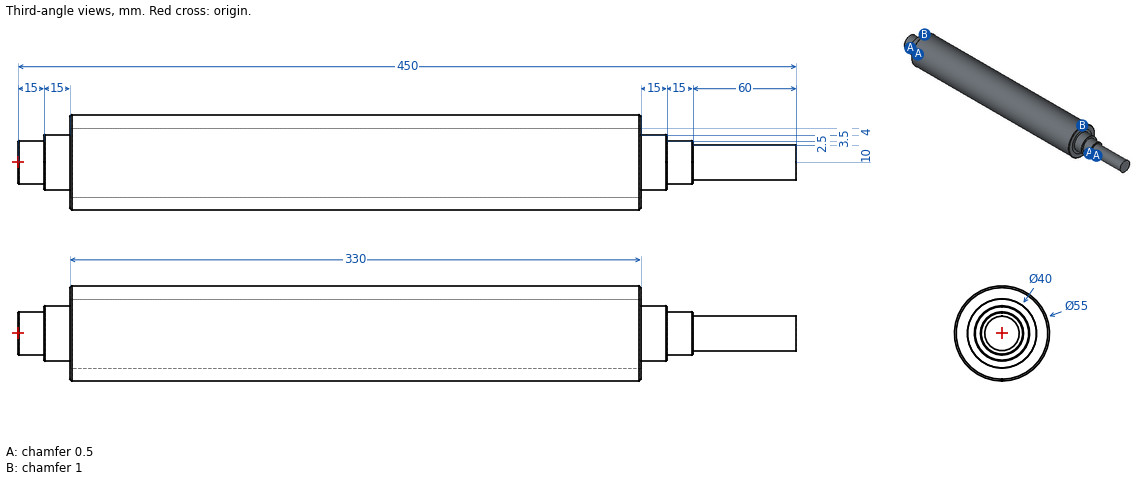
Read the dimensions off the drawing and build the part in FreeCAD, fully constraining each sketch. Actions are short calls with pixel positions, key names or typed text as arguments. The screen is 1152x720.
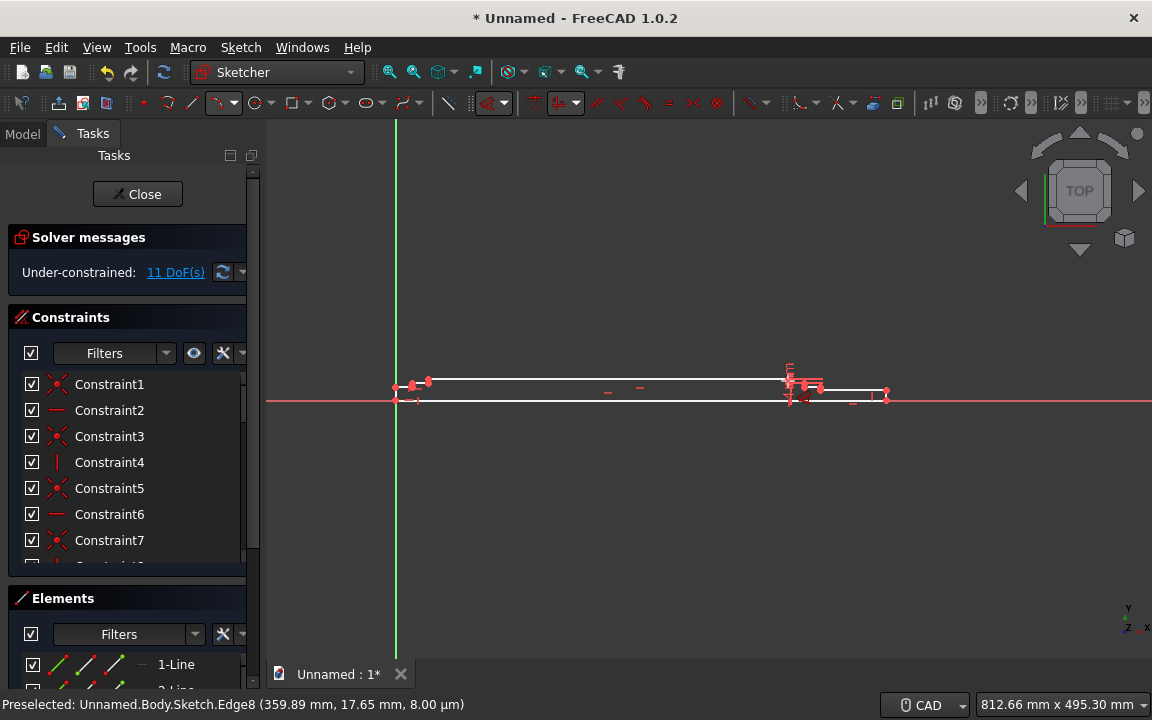
scroll(428, 380, up, 12)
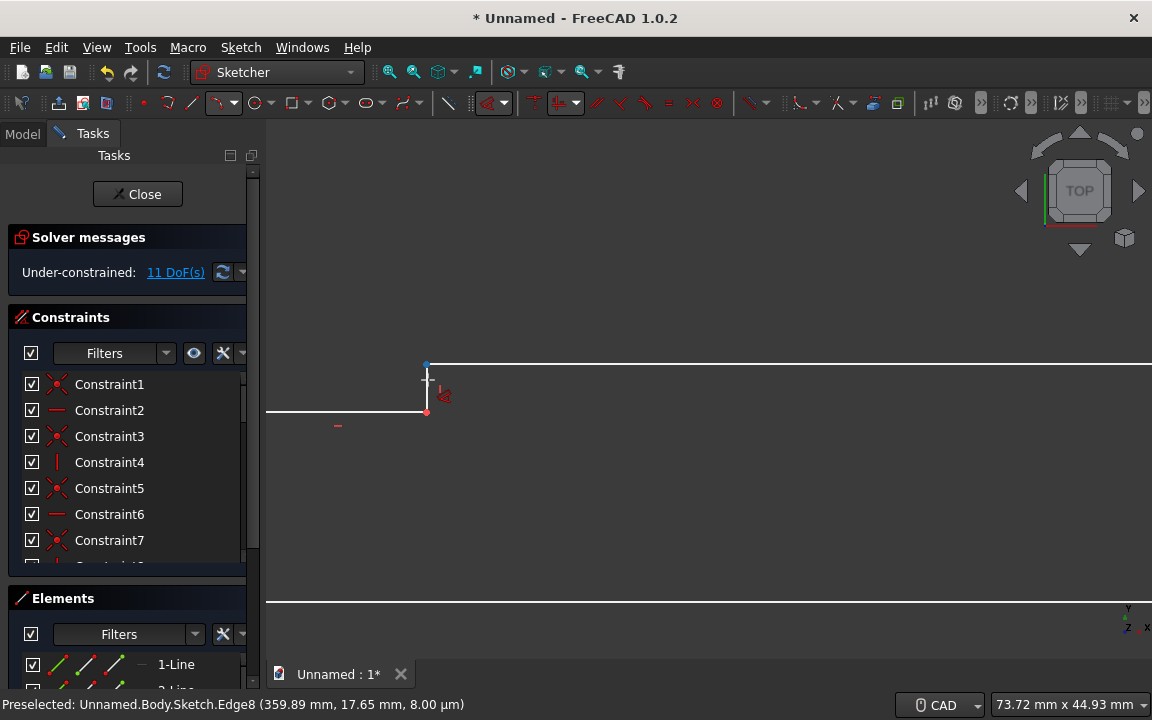
click(427, 379)
click(393, 388)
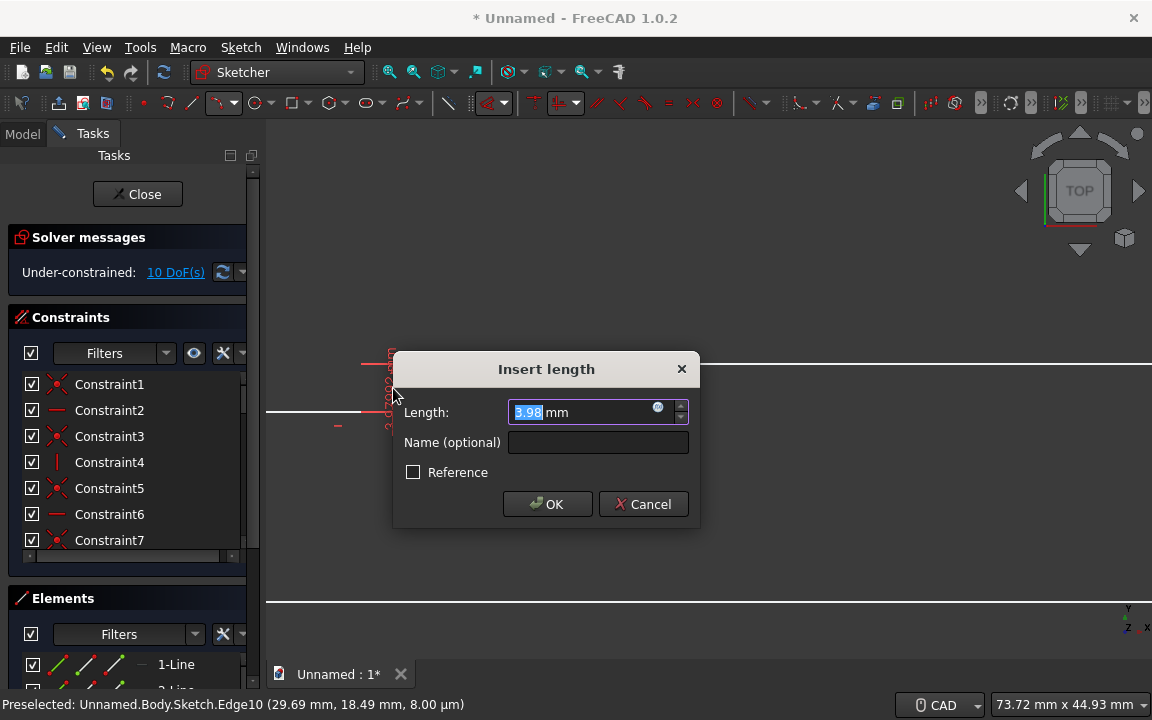
text(4)
key(Return)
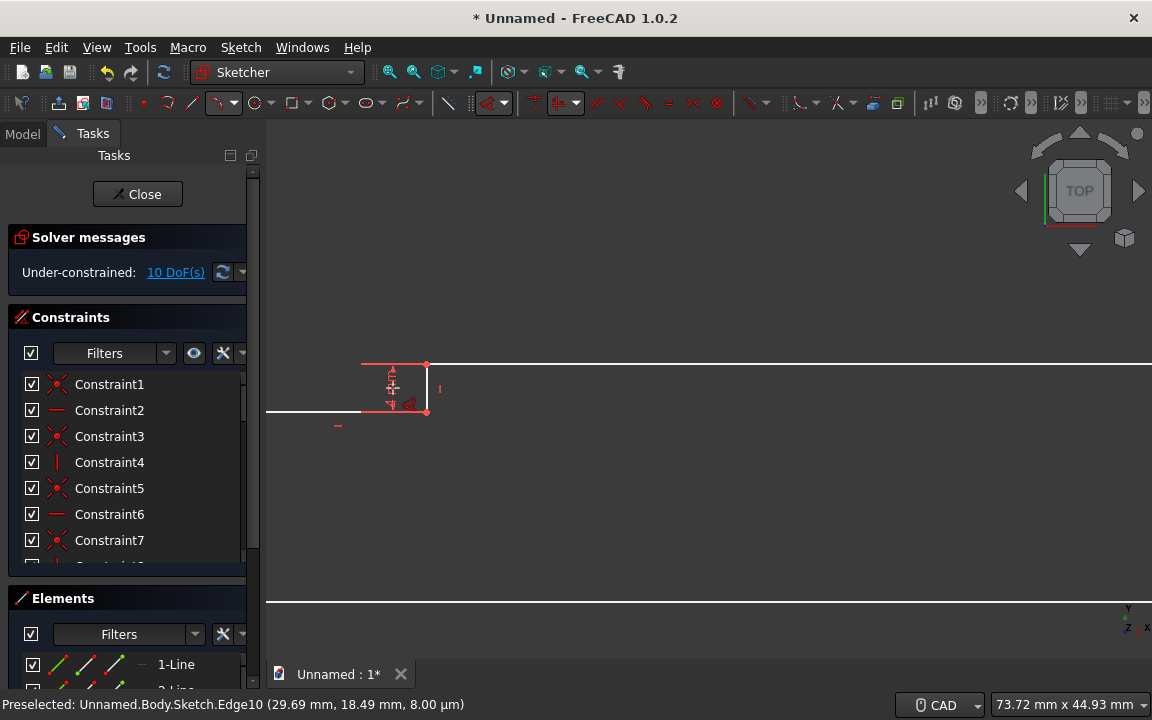
scroll(428, 380, down, 12)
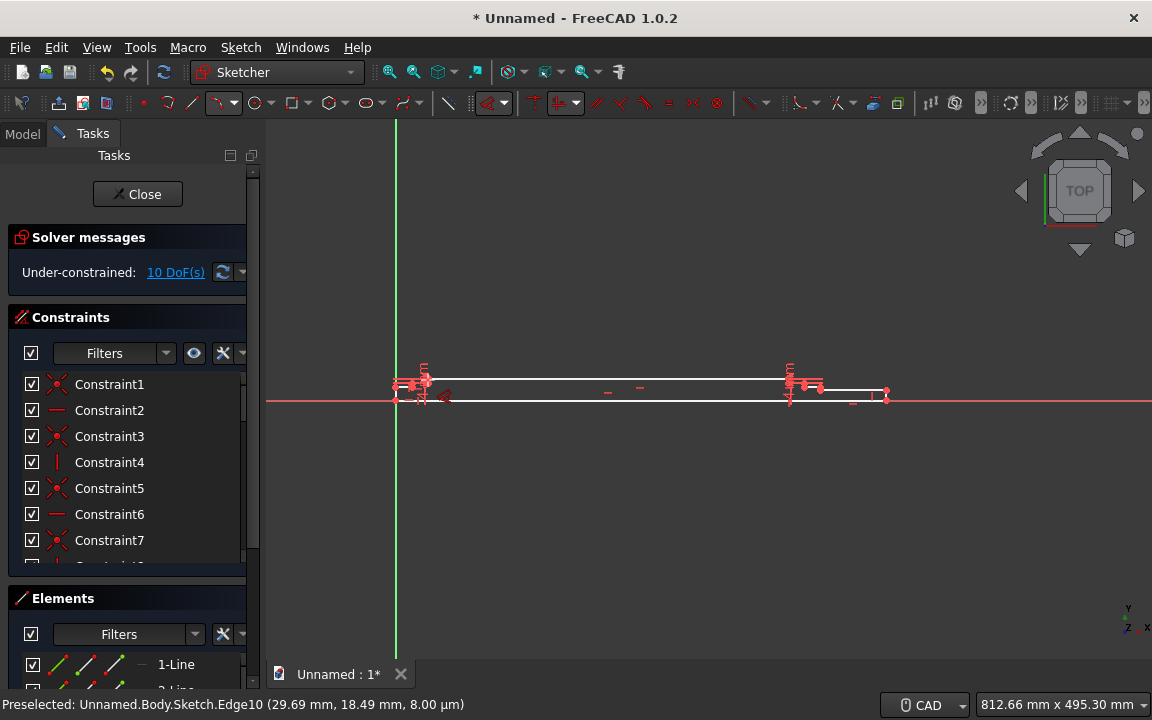
scroll(886, 397, up, 8)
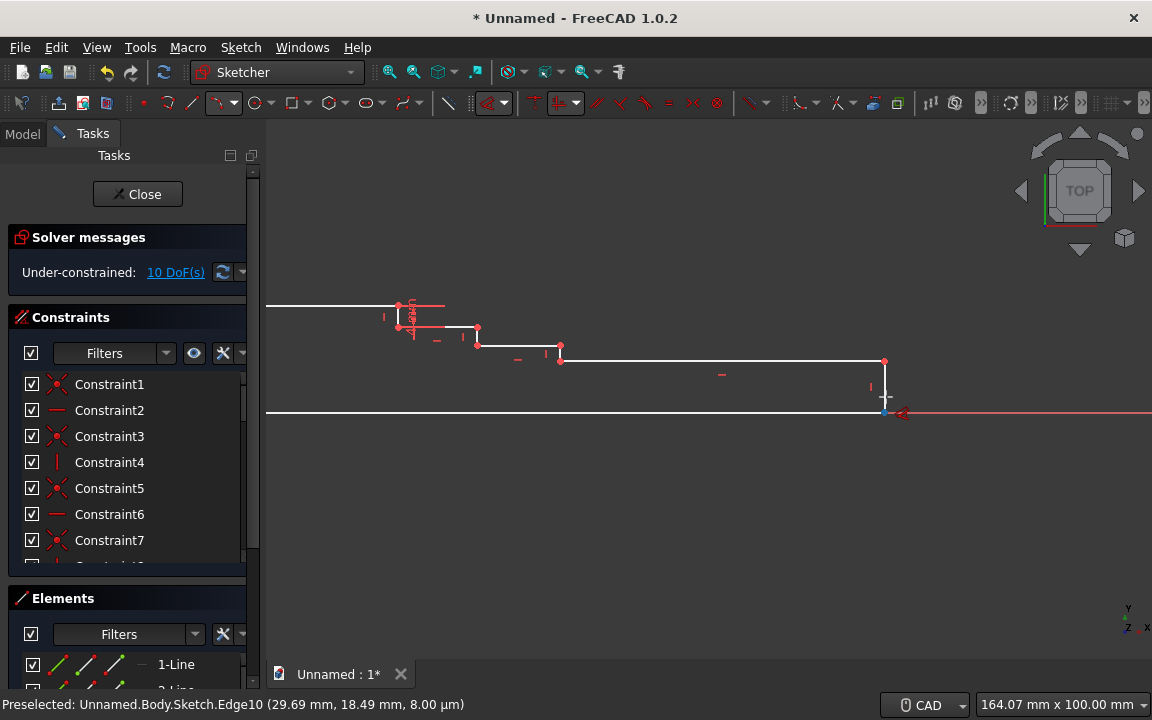
click(885, 397)
click(919, 387)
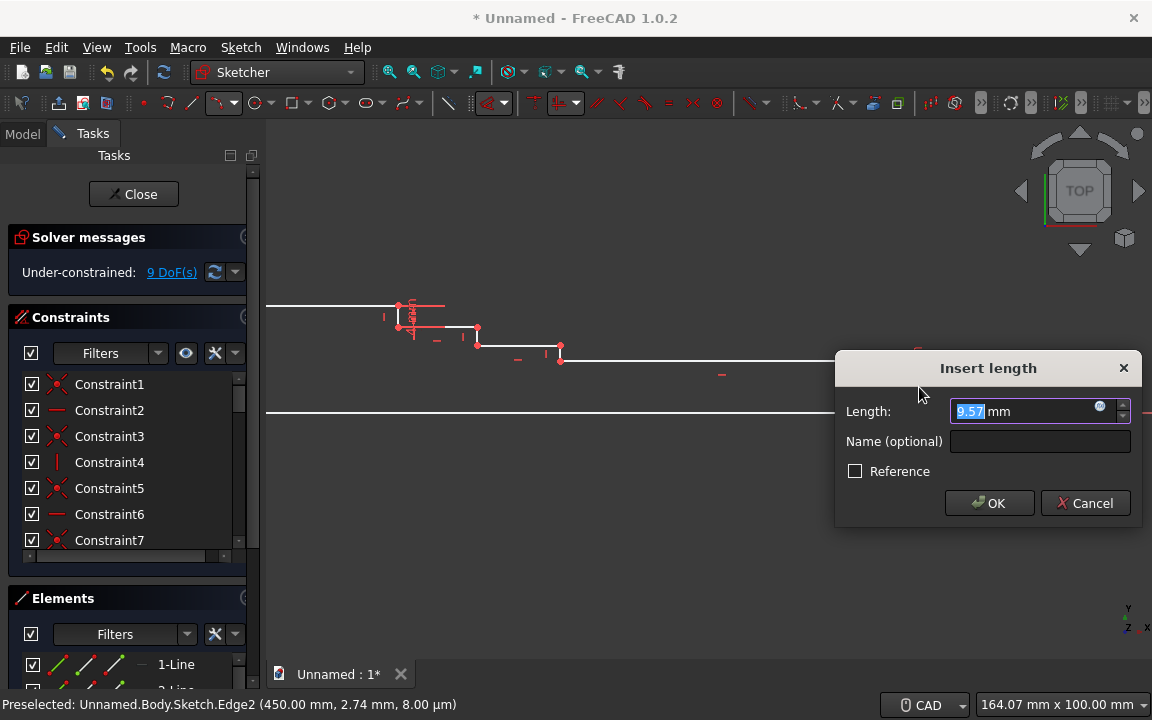
text(10)
key(Return)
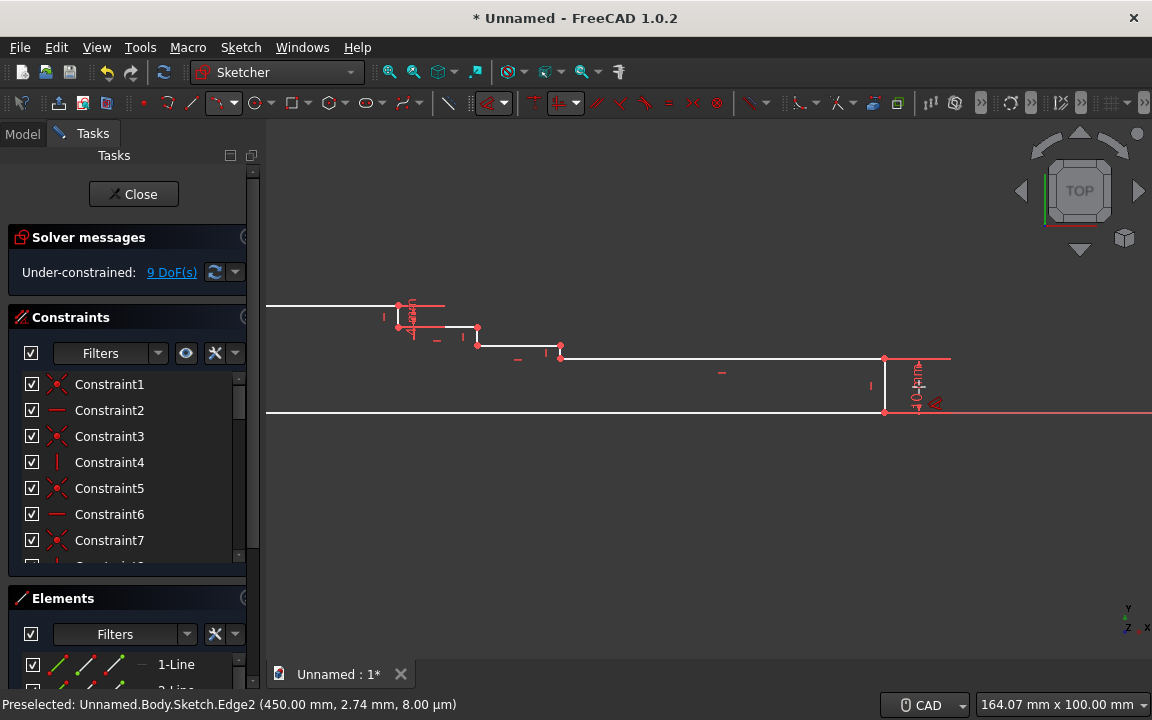
scroll(886, 397, down, 8)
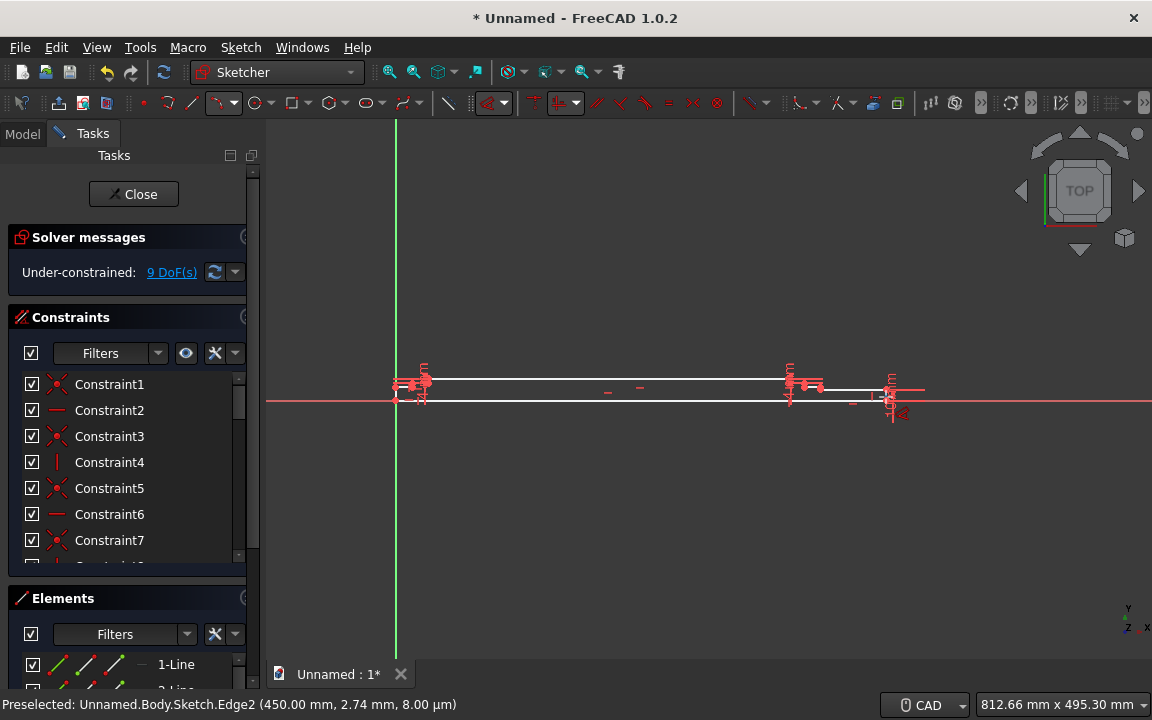
scroll(867, 390, up, 2)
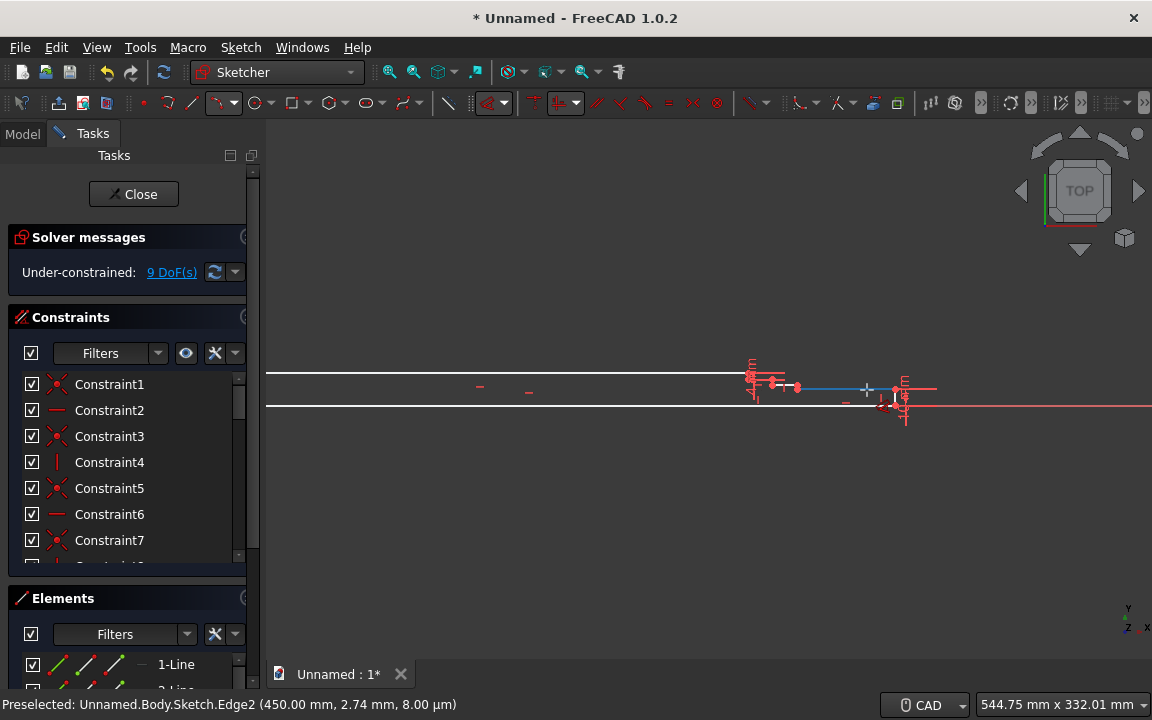
click(866, 389)
click(847, 423)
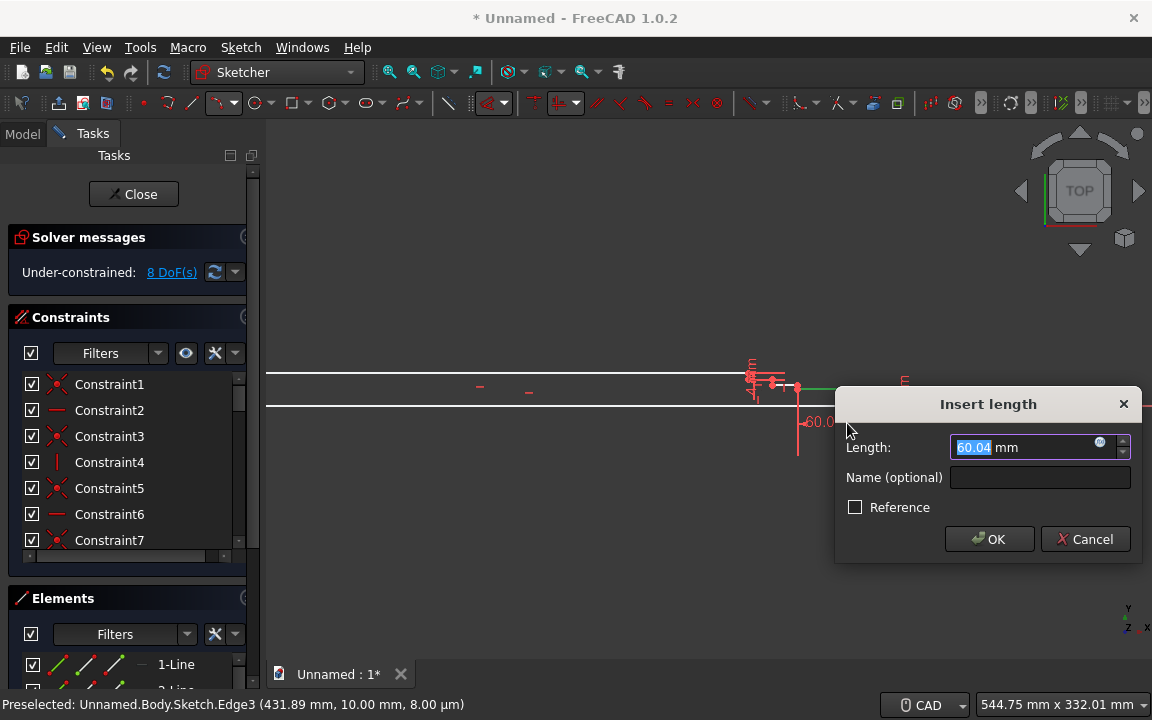
text(60)
key(Return)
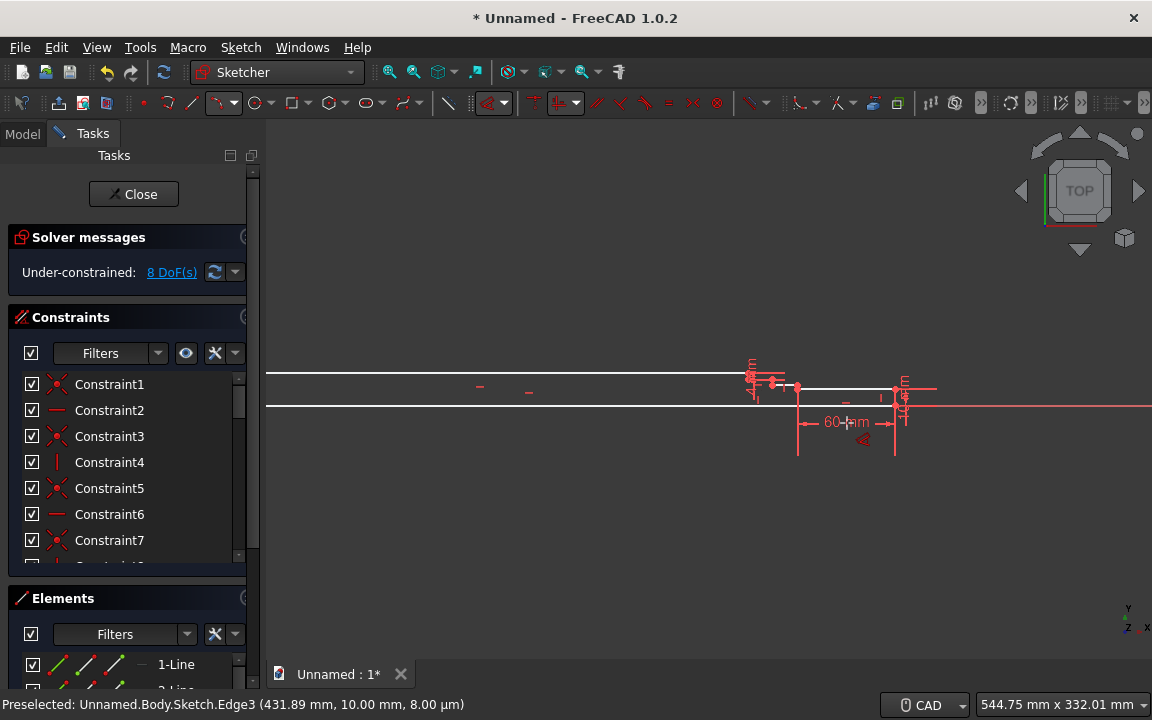
scroll(788, 385, up, 3)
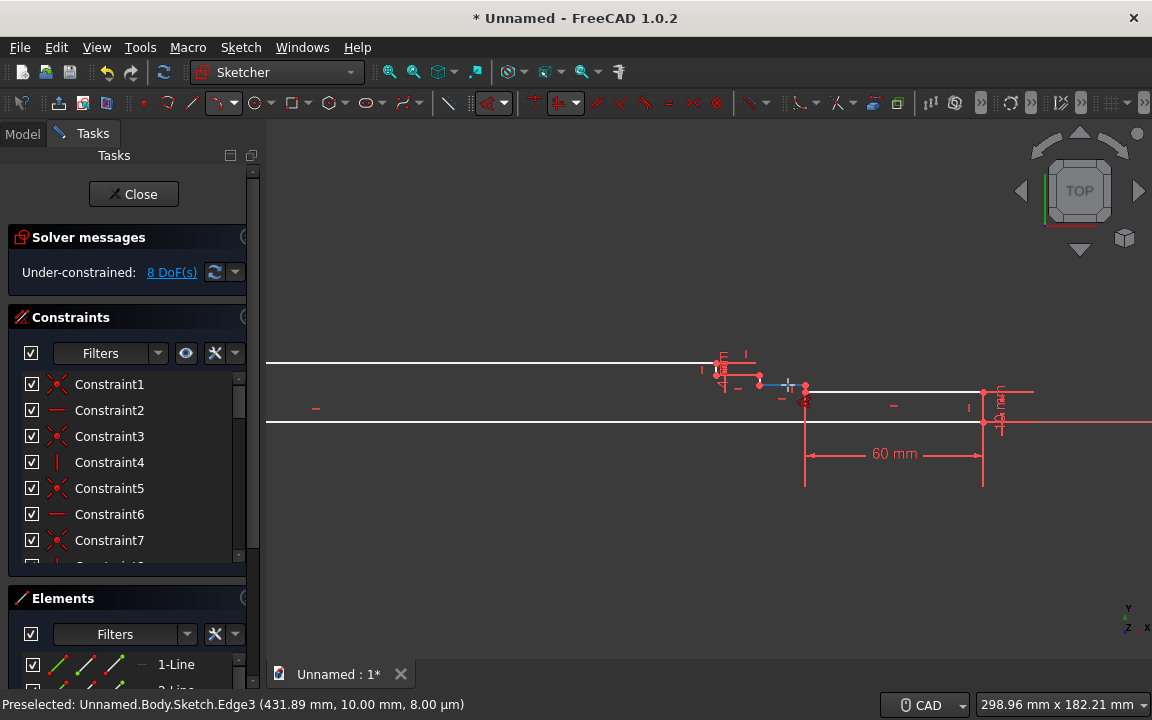
click(787, 385)
click(799, 351)